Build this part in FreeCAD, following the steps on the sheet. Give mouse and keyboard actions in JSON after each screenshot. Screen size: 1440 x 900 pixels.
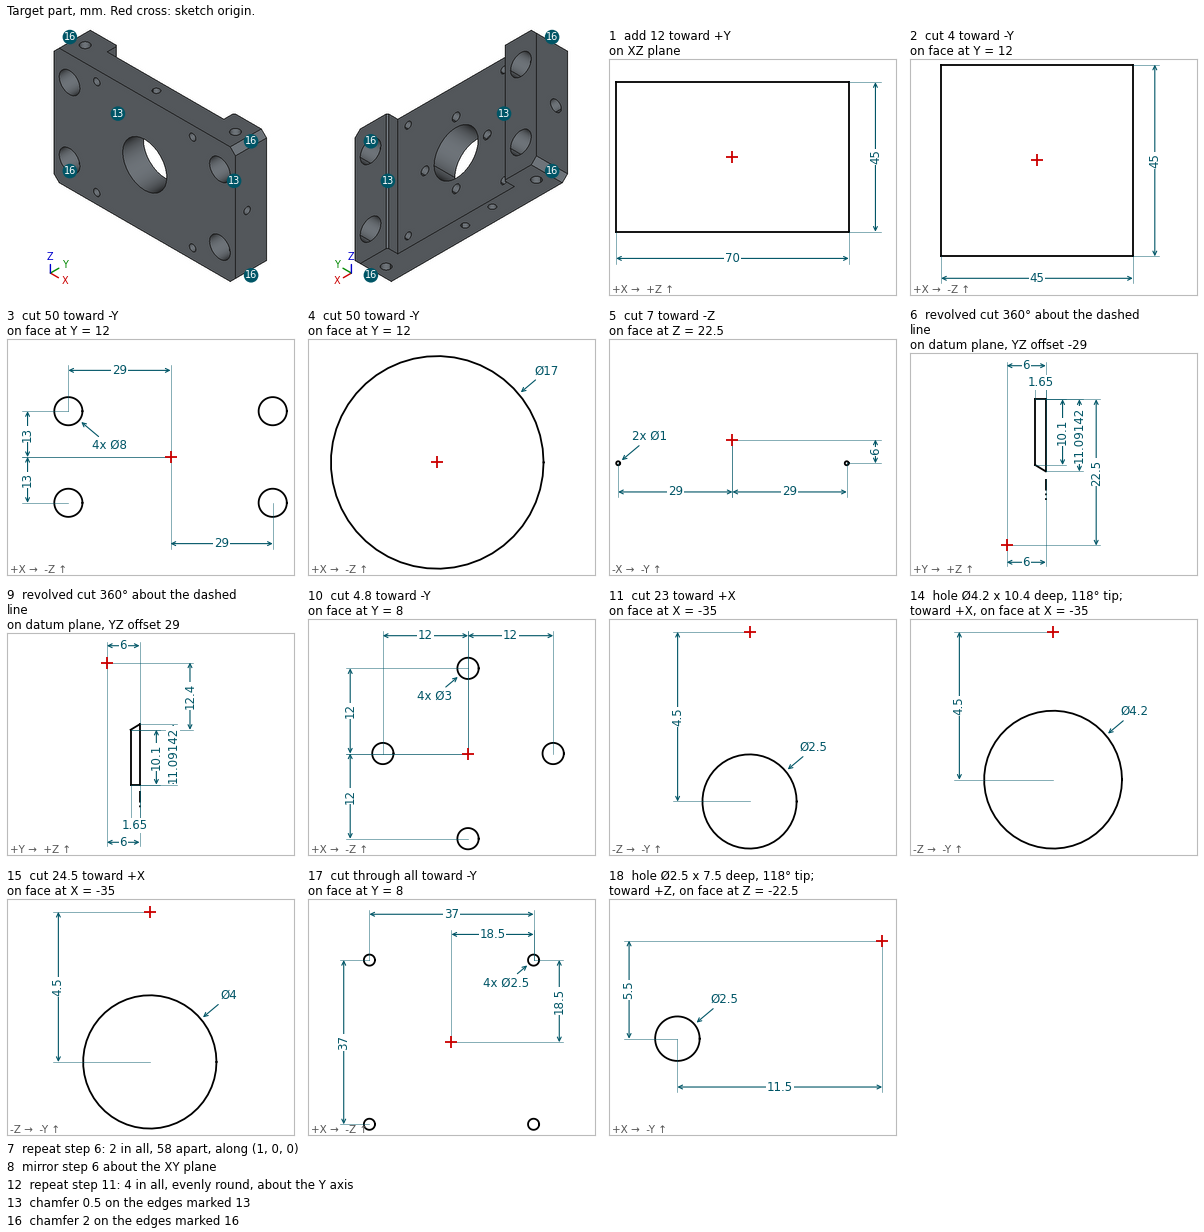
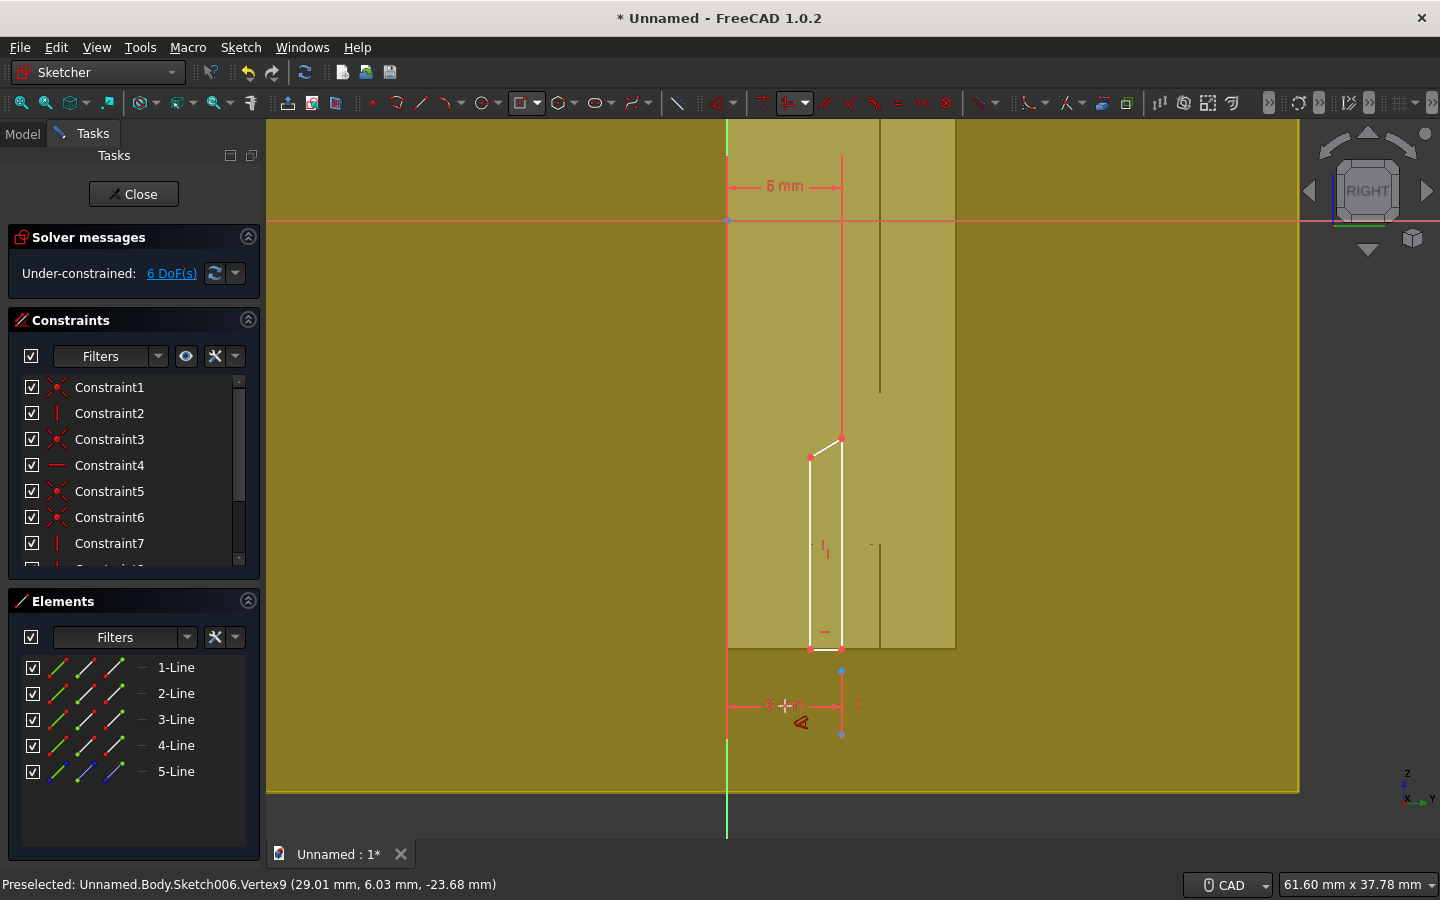
{"action": "left_click", "coordinate": [810, 516]}
{"action": "left_click", "coordinate": [776, 554]}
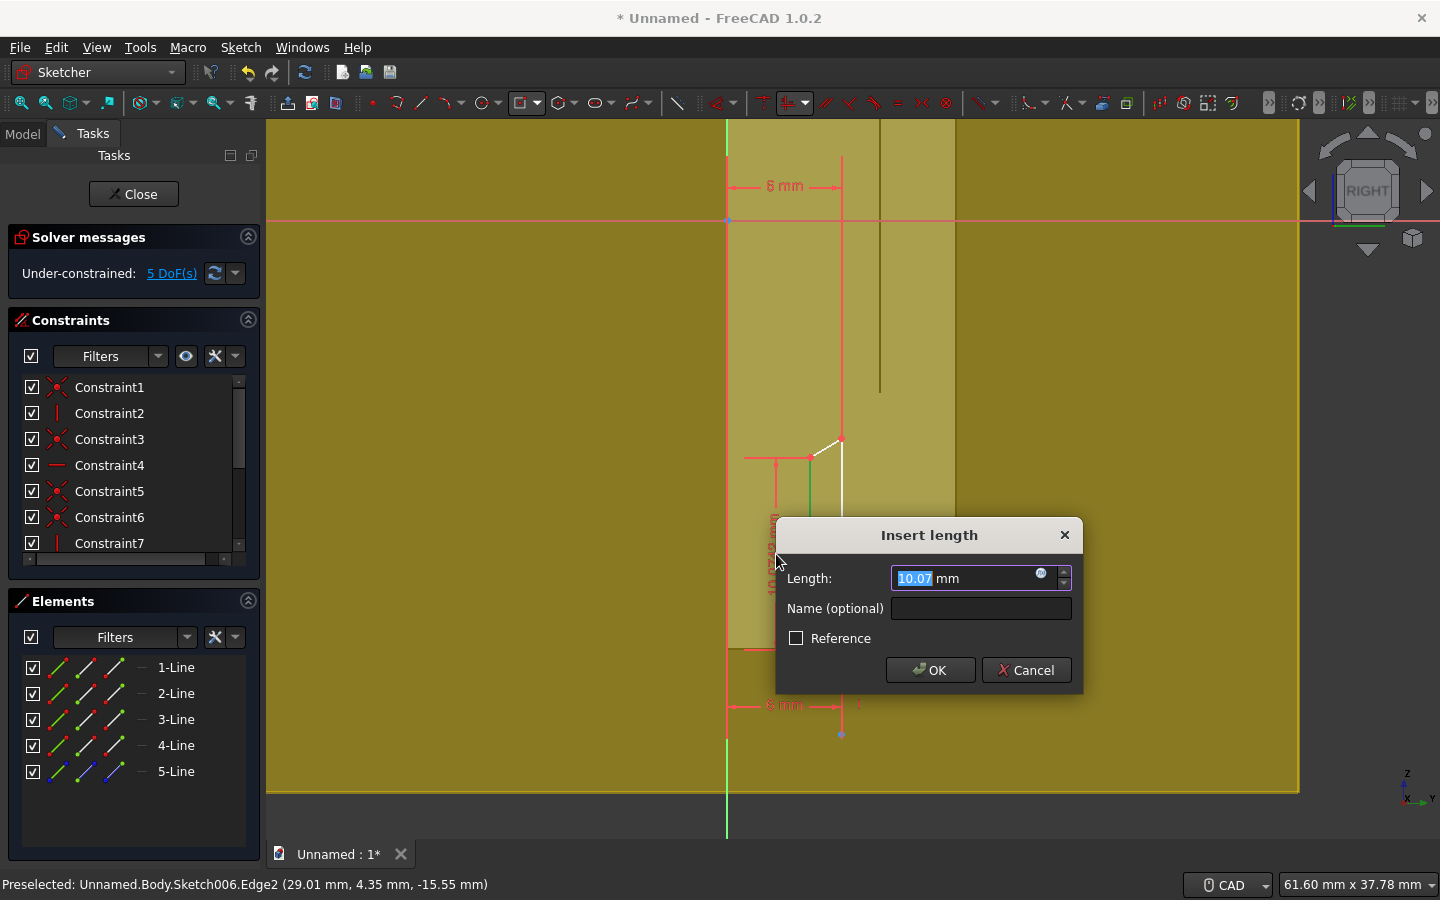
{"action": "type", "text": "10.1"}
{"action": "key", "text": "Return"}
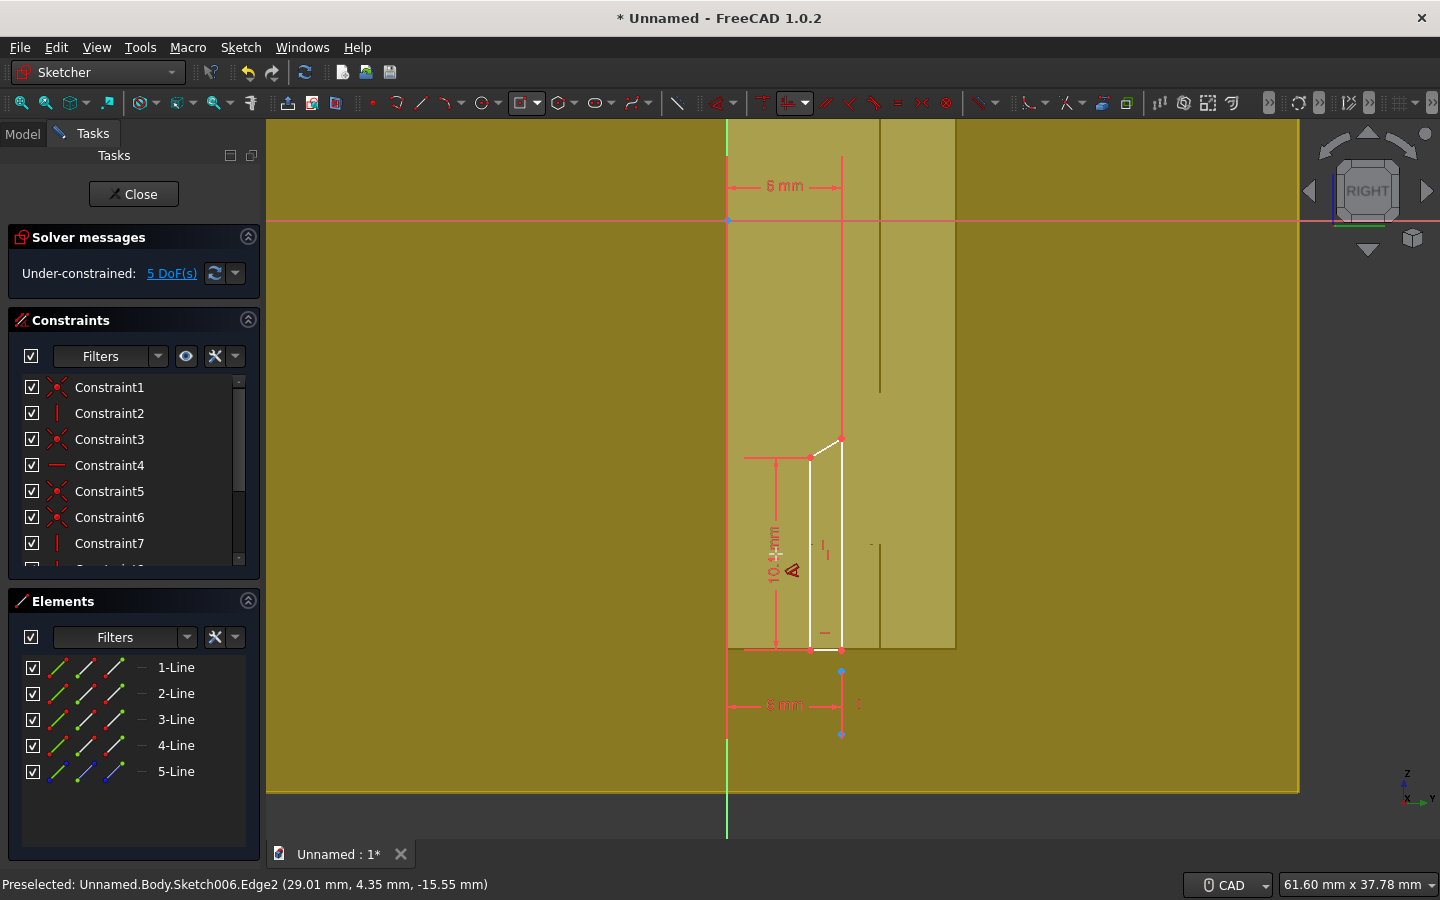
{"action": "scroll", "coordinate": [819, 650], "scroll_direction": "up", "scroll_amount": 2}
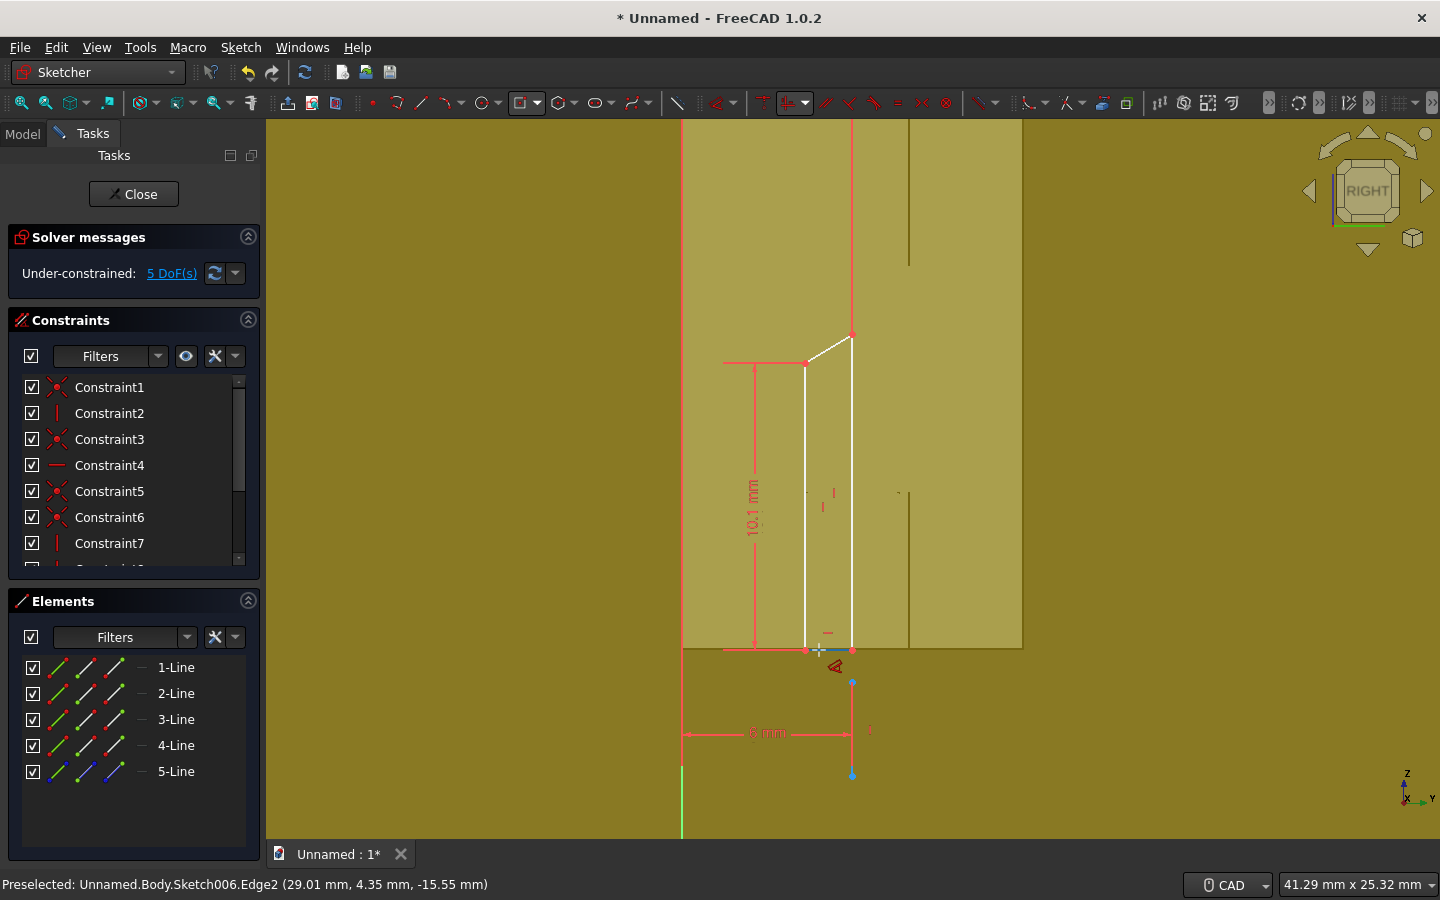
{"action": "left_click", "coordinate": [819, 650]}
{"action": "left_click", "coordinate": [829, 684]}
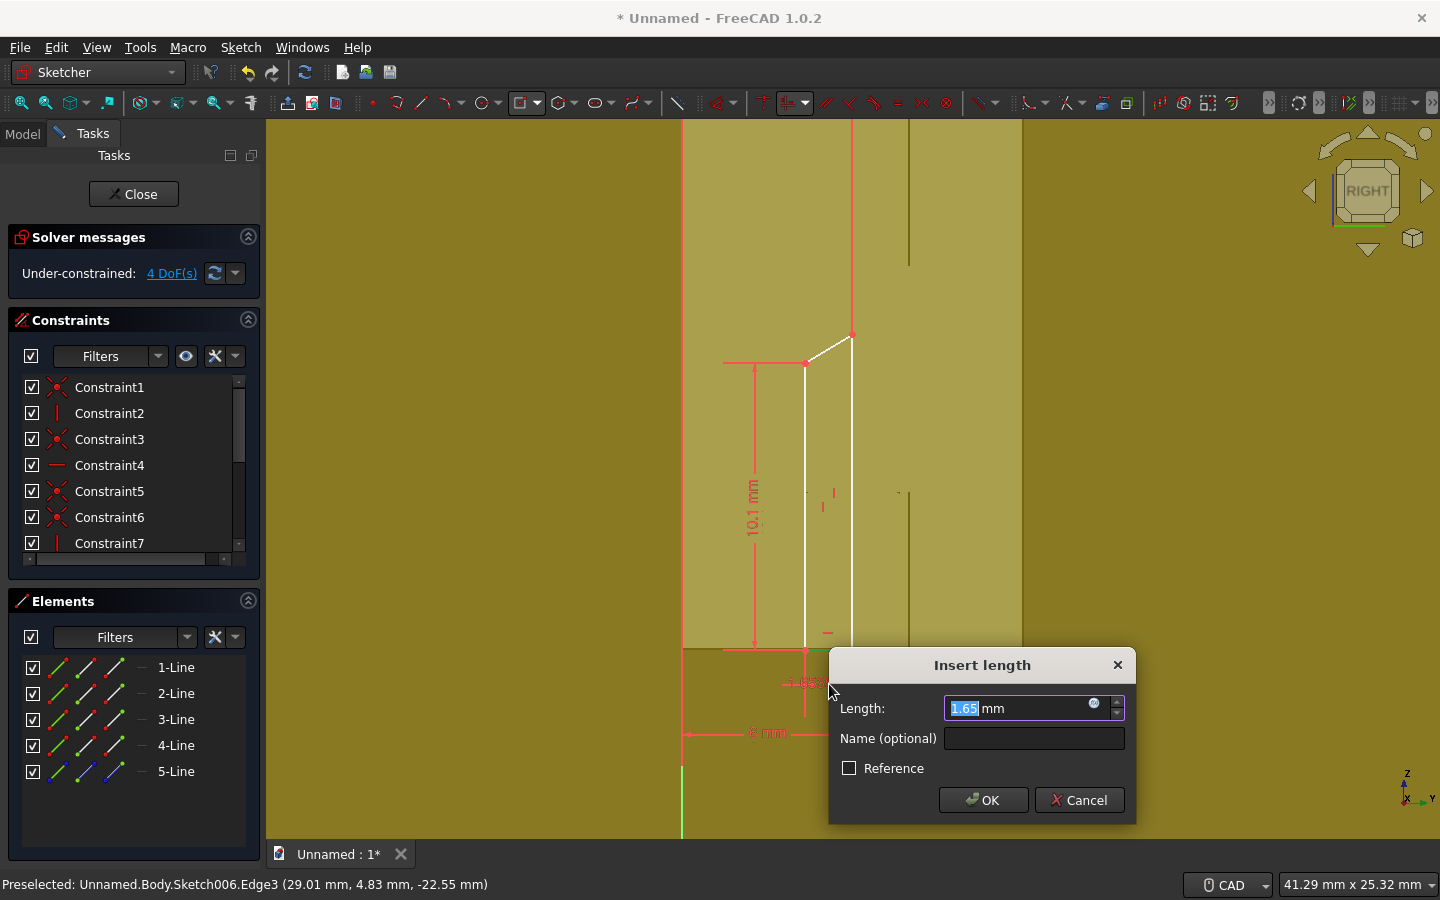
{"action": "type", "text": "1.65"}
{"action": "key", "text": "Return"}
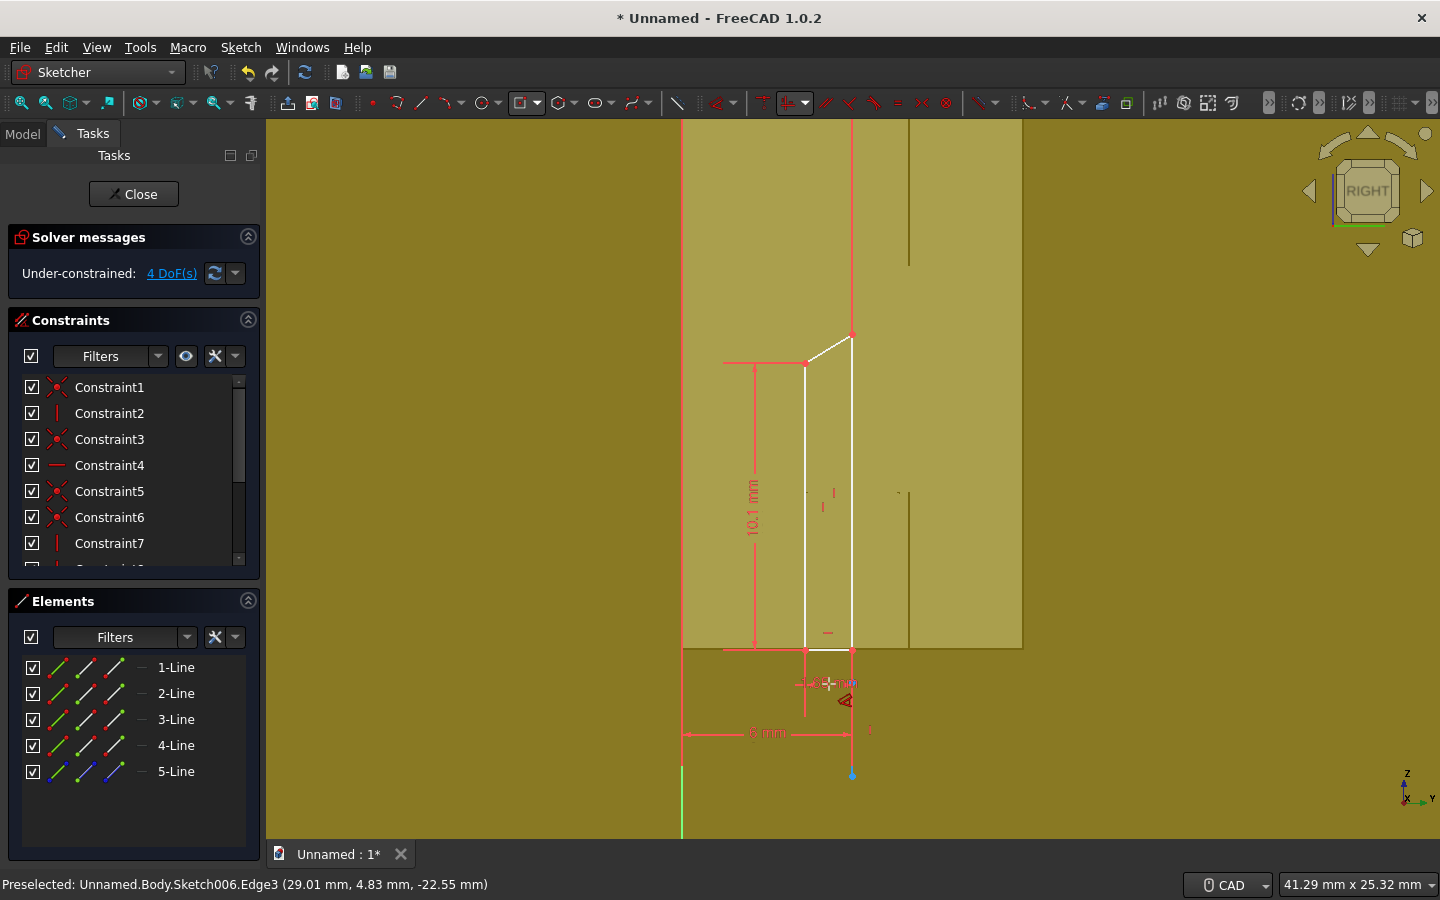
{"action": "left_click", "coordinate": [805, 363]}
{"action": "left_click", "coordinate": [648, 255]}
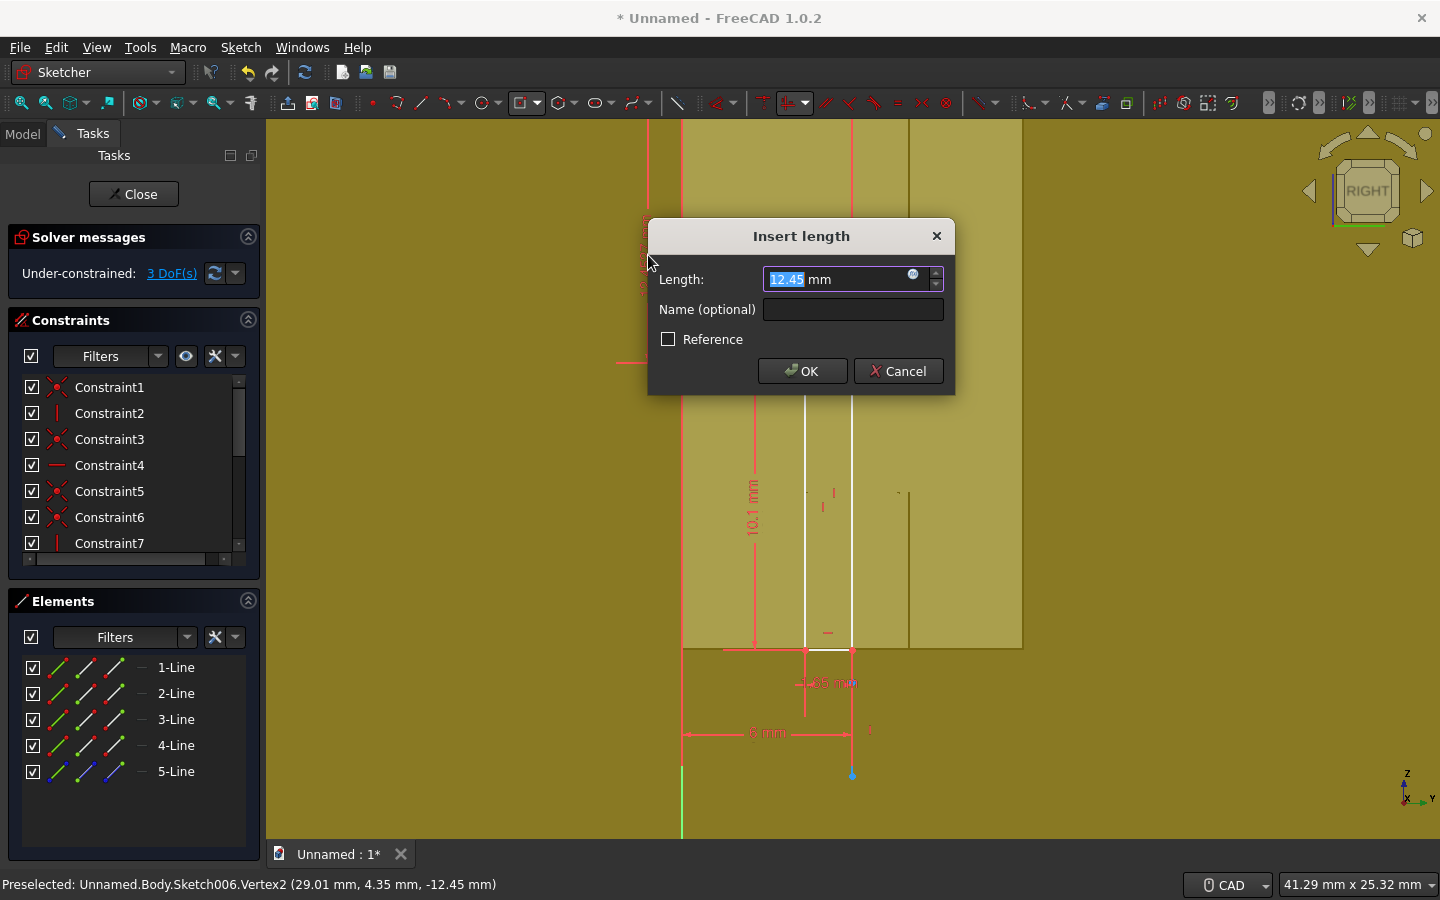
{"action": "type", "text": "12.4"}
{"action": "key", "text": "Return"}